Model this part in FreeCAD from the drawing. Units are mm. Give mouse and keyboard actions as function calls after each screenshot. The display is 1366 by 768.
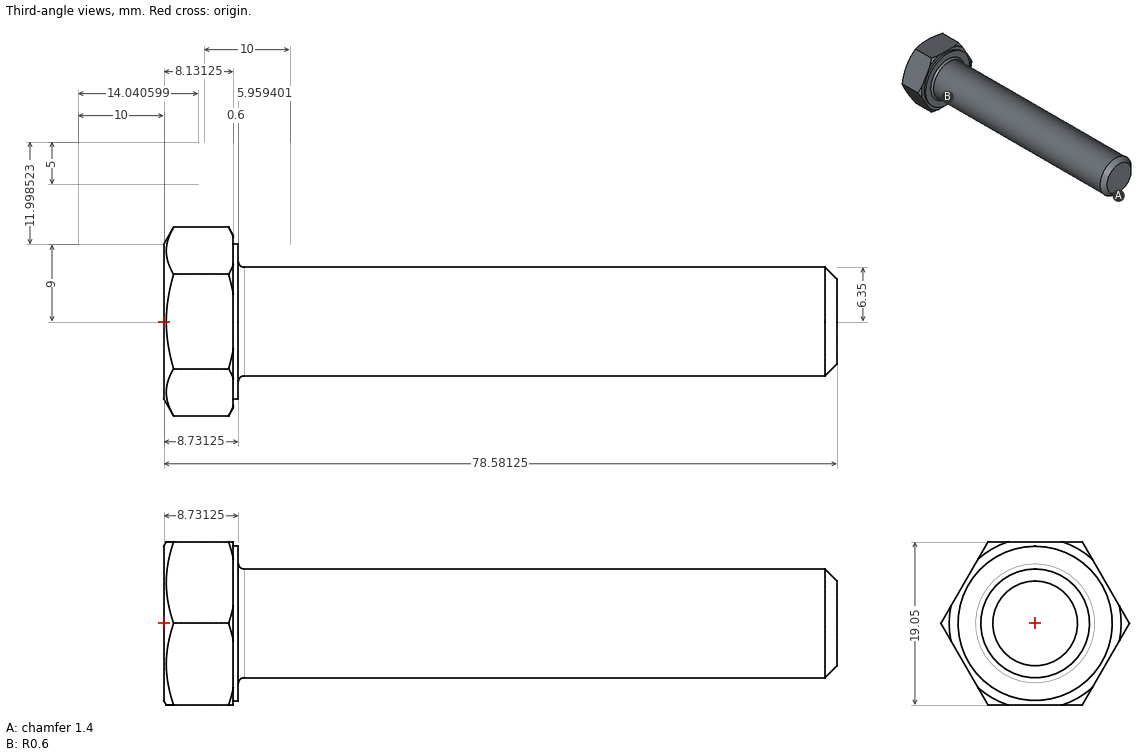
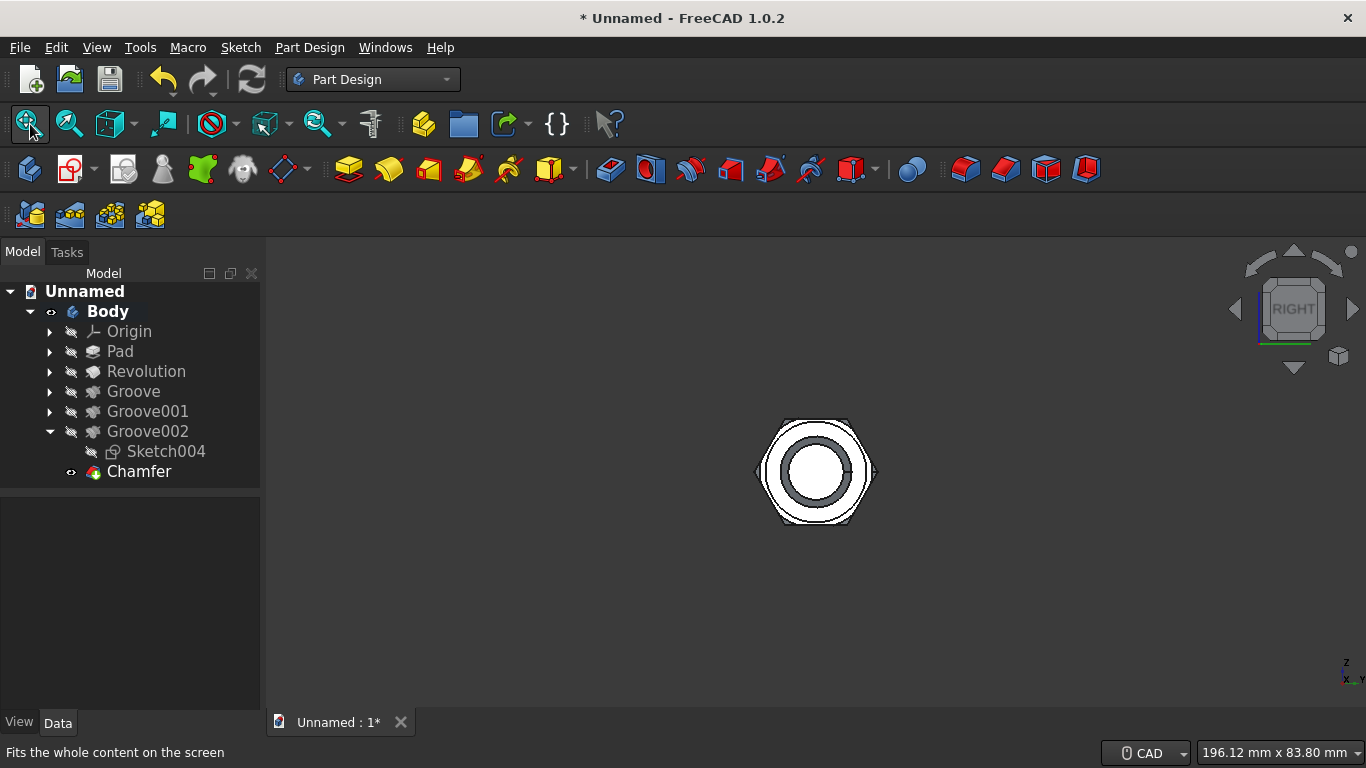
click(30, 124)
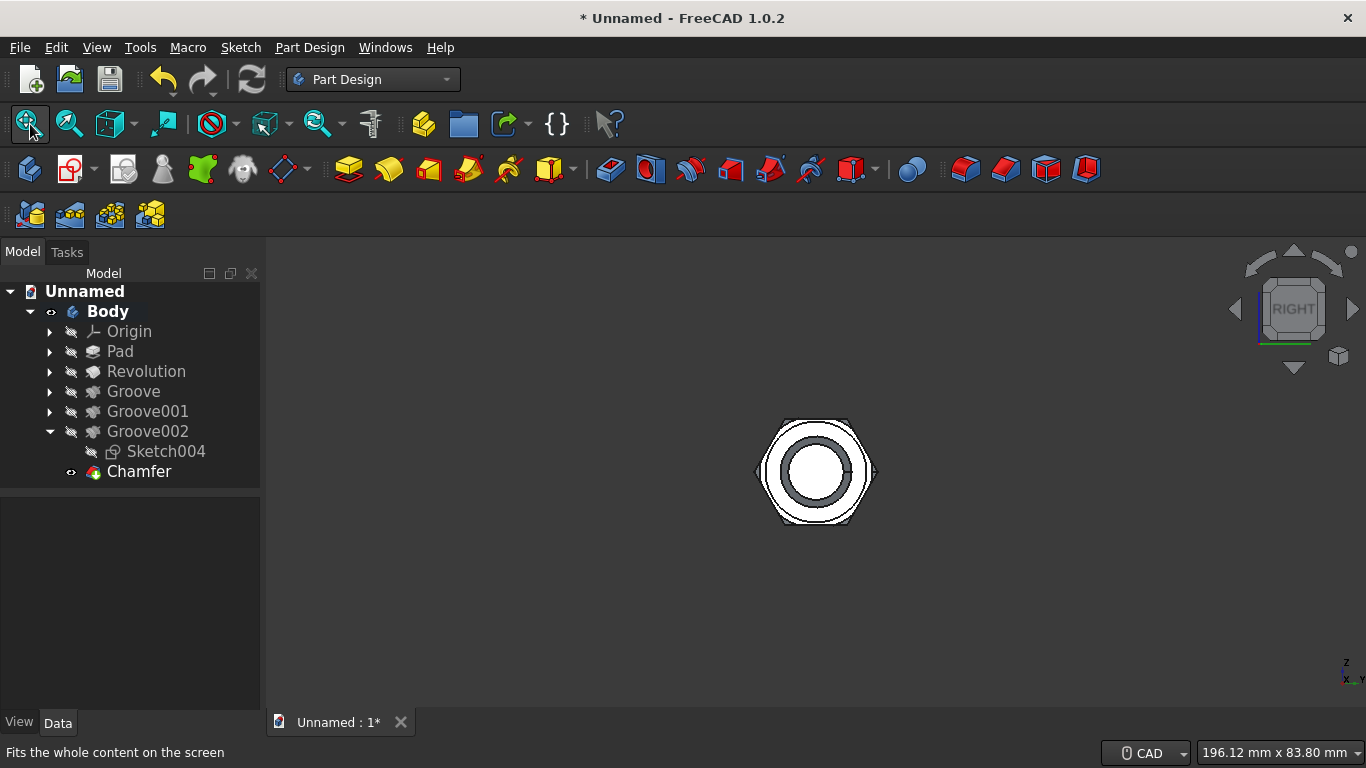
key(5)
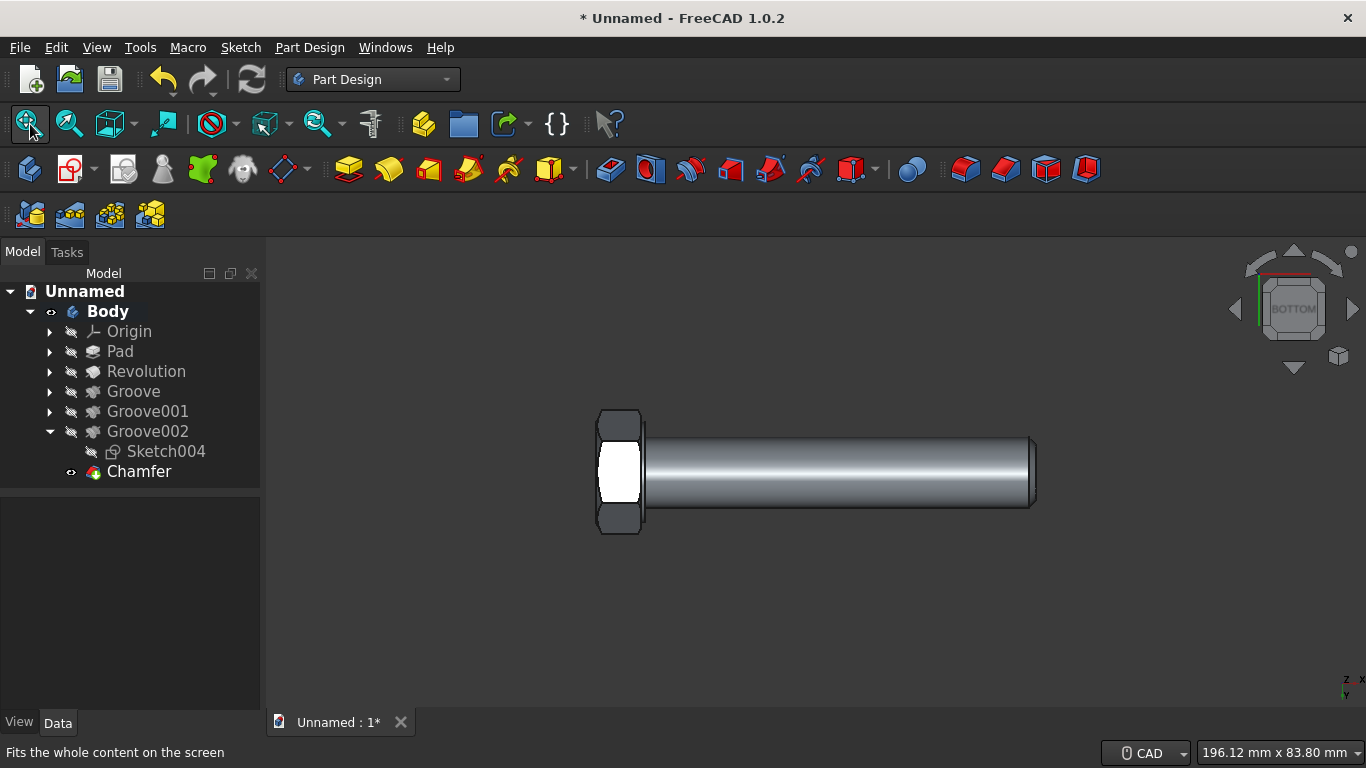
click(30, 124)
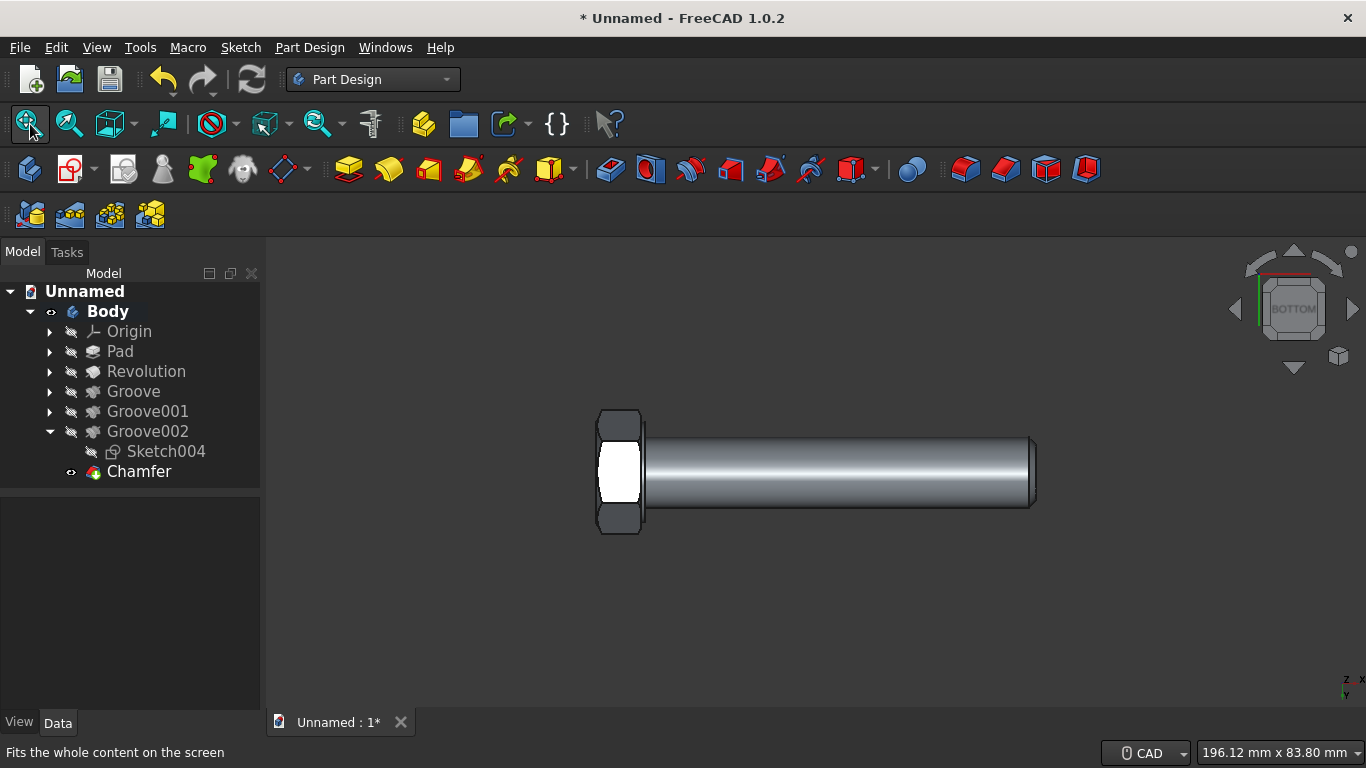
key(4)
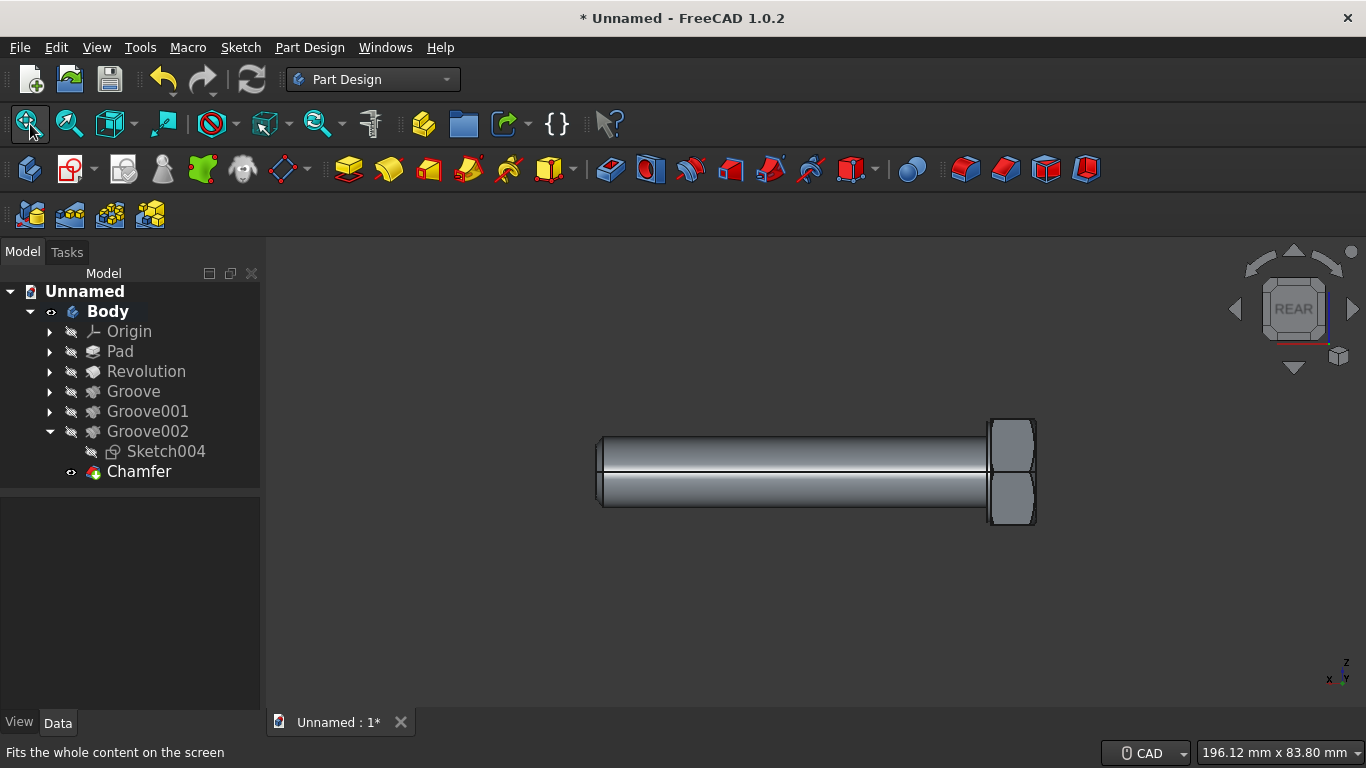
click(30, 124)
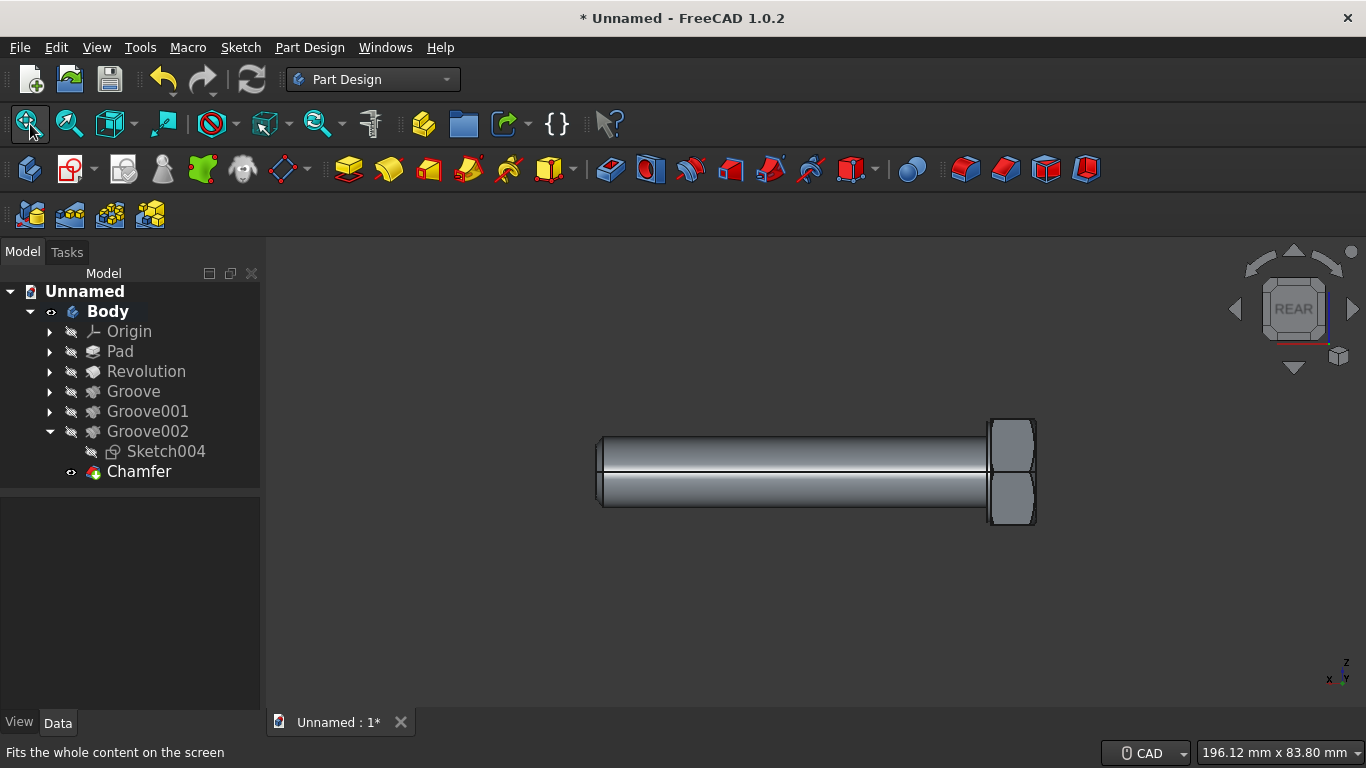
key(6)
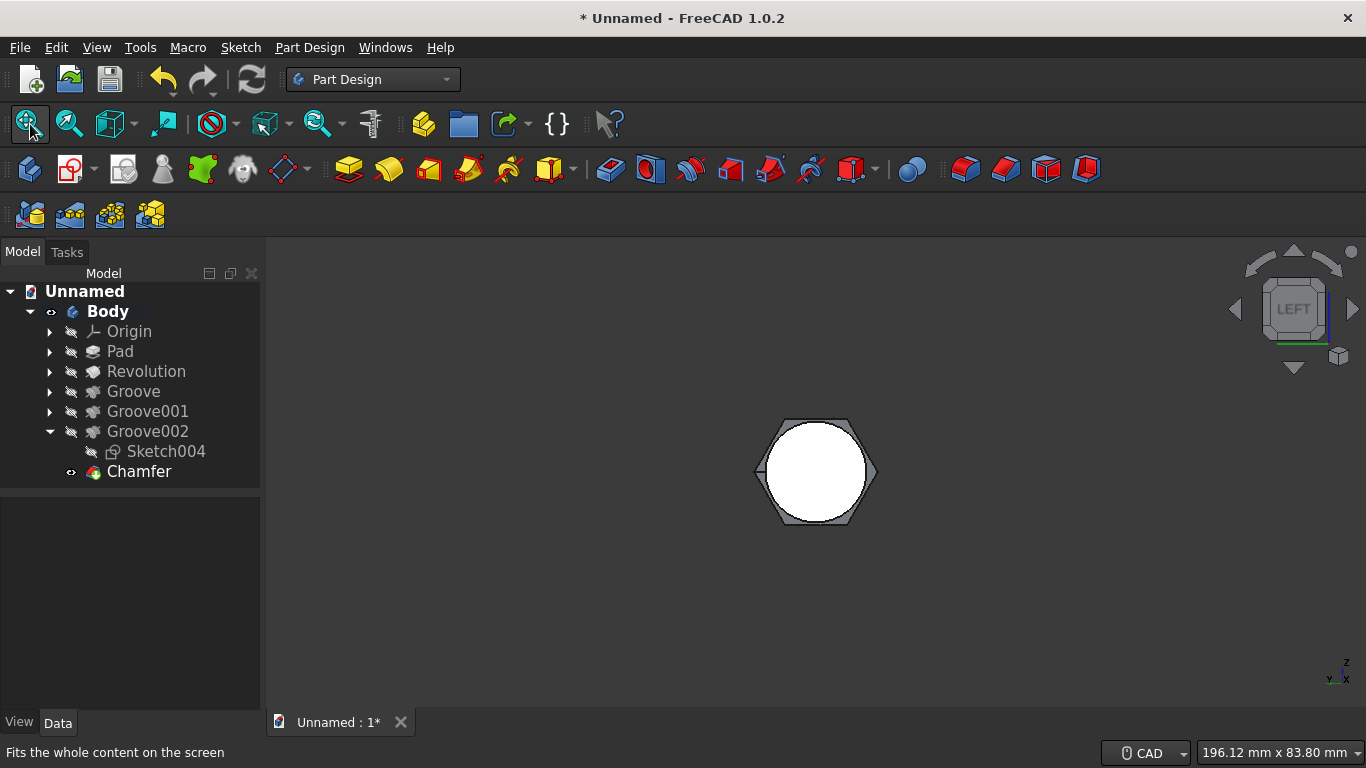
click(30, 124)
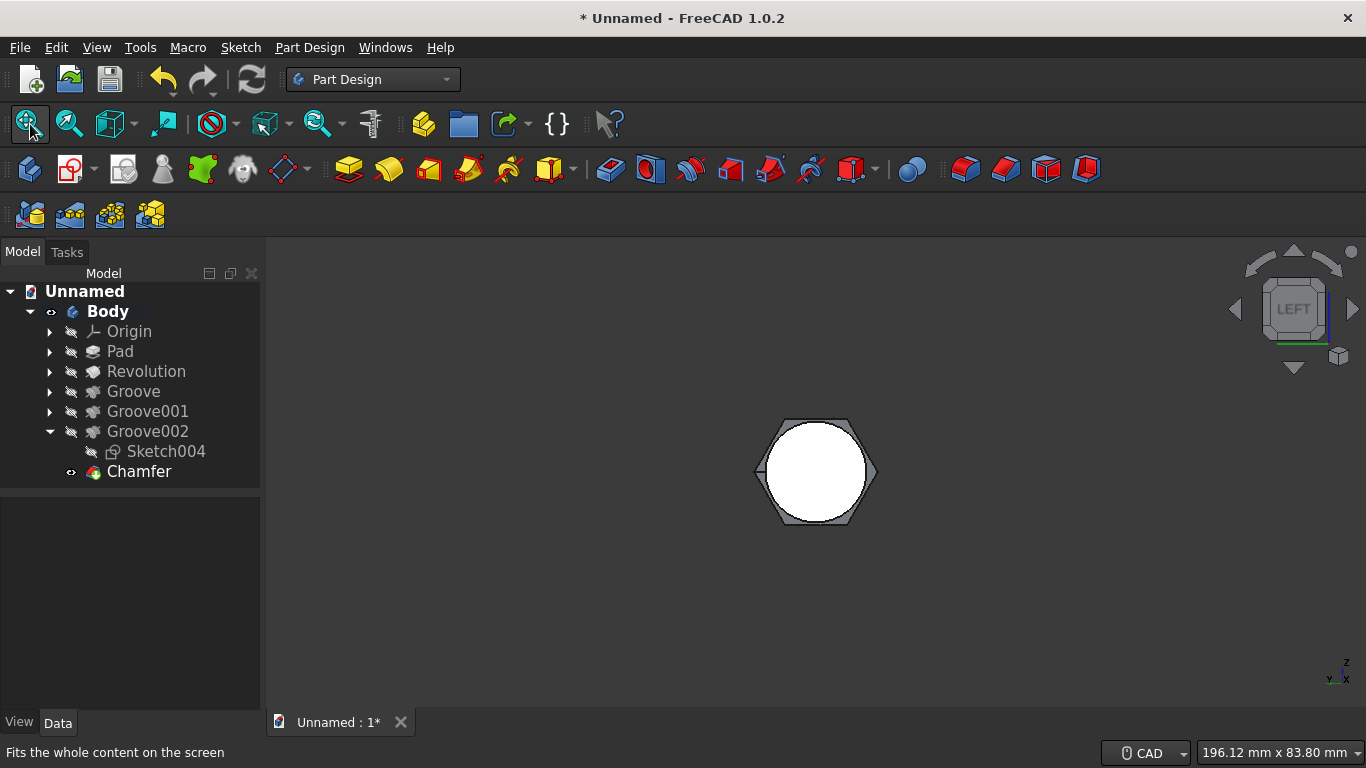
key(v)
key(3)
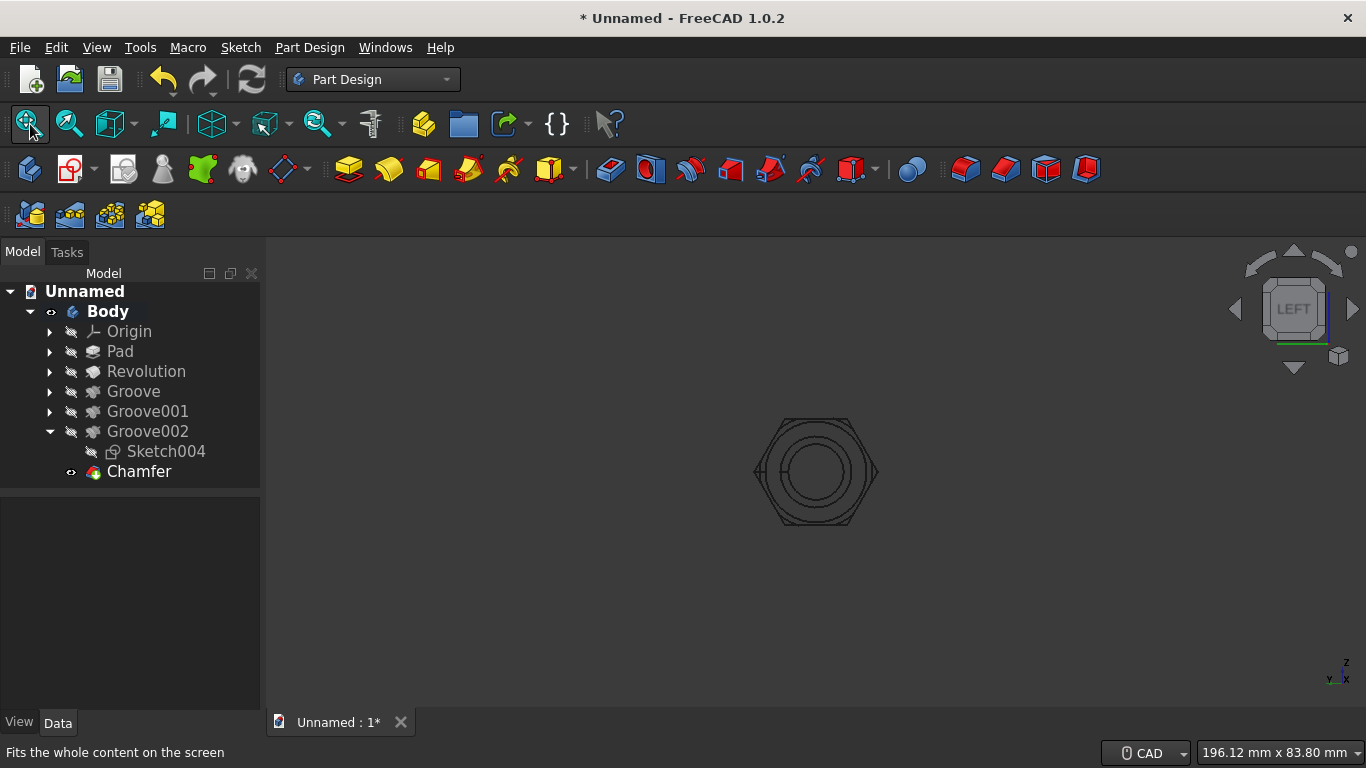
key(0)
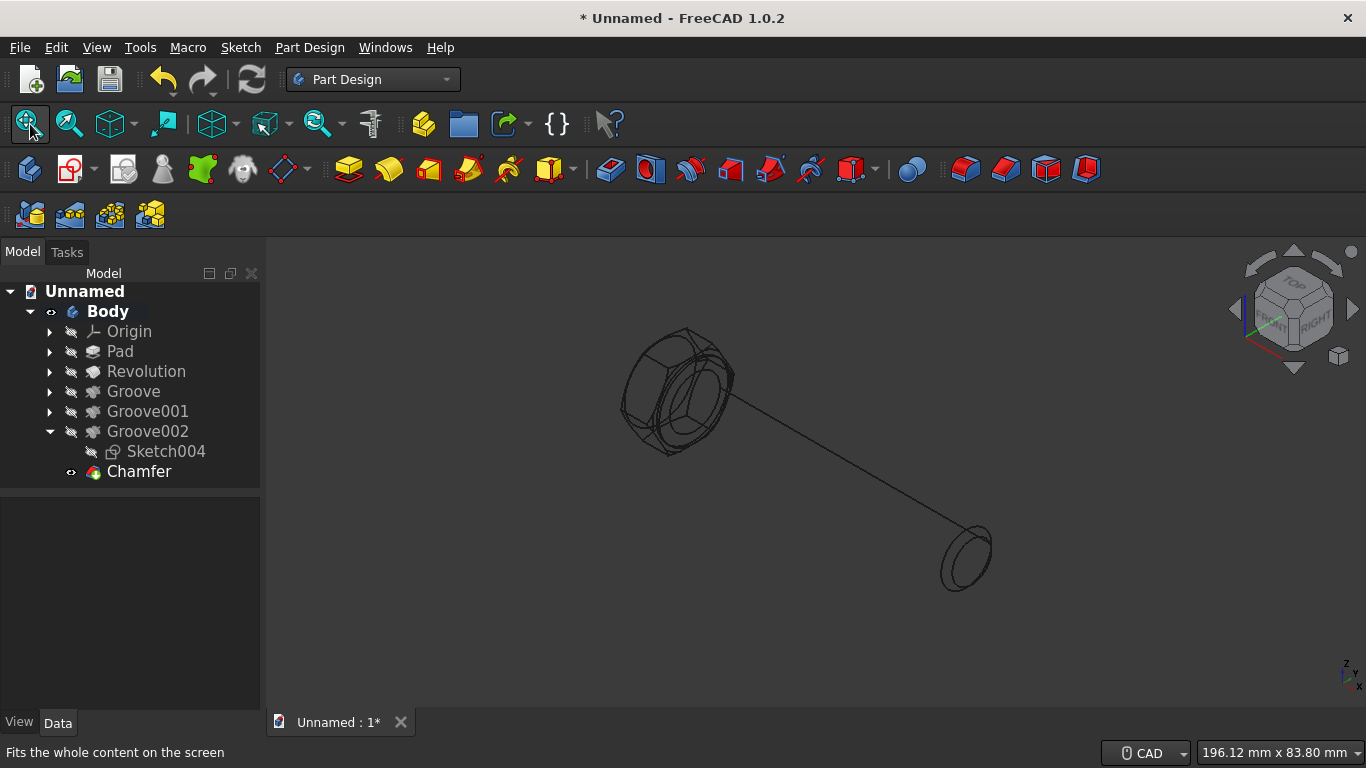
click(670, 416)